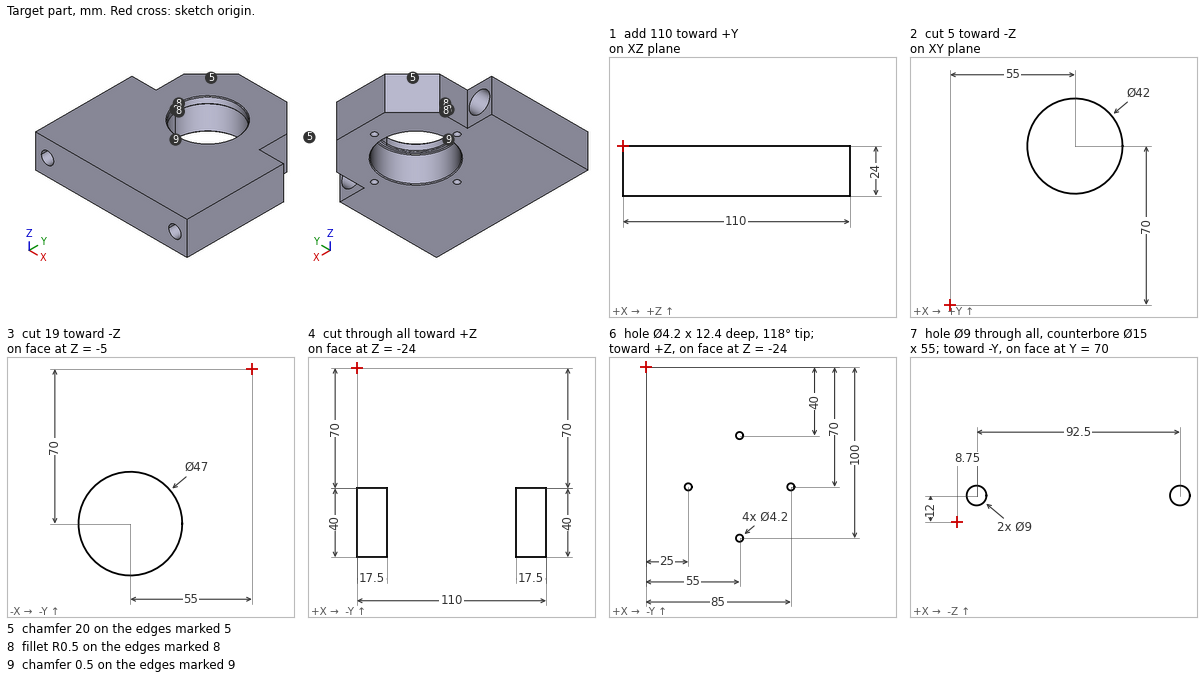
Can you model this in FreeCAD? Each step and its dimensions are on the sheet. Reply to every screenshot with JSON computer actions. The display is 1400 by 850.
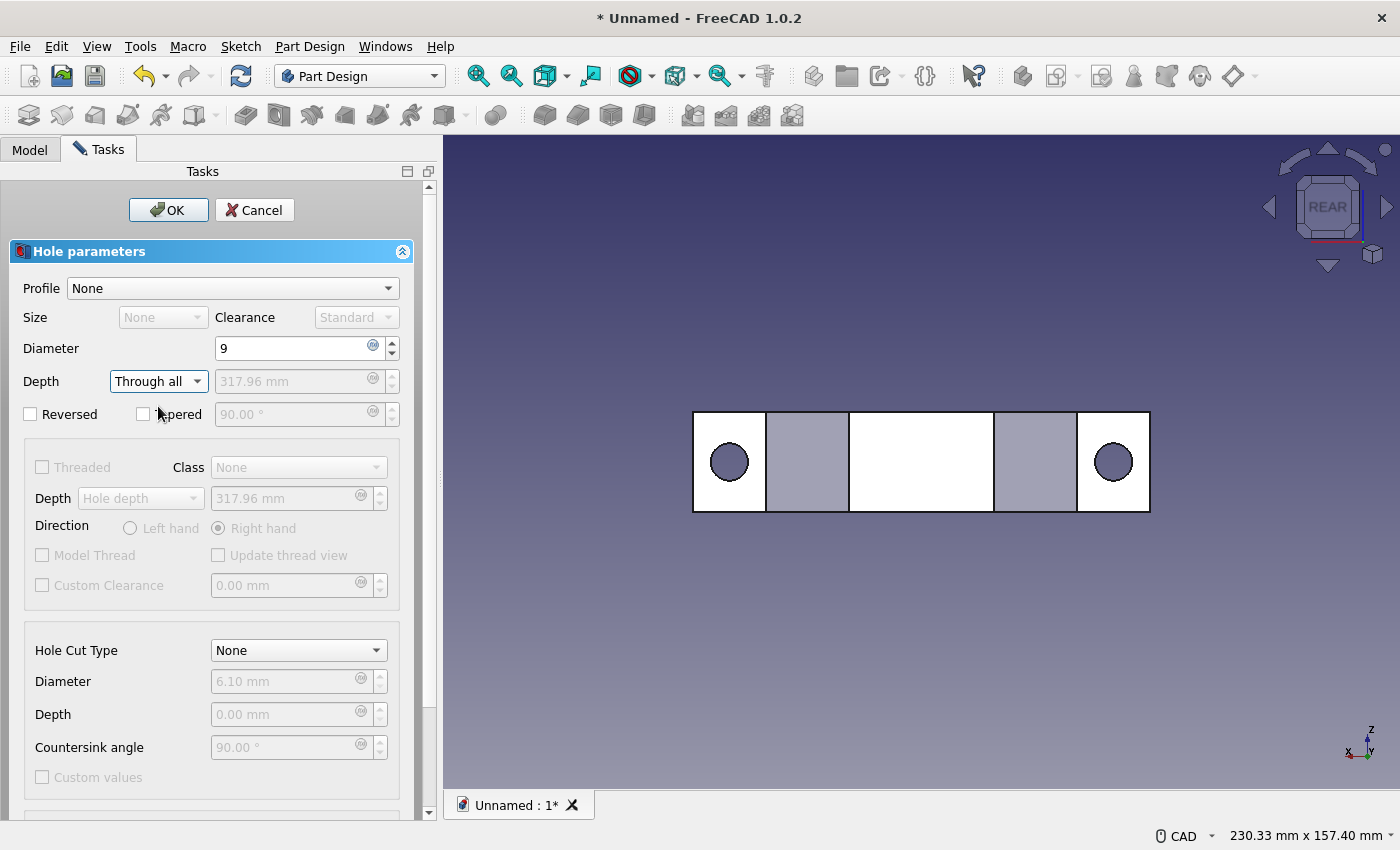
{"action": "left_click", "coordinate": [300, 650]}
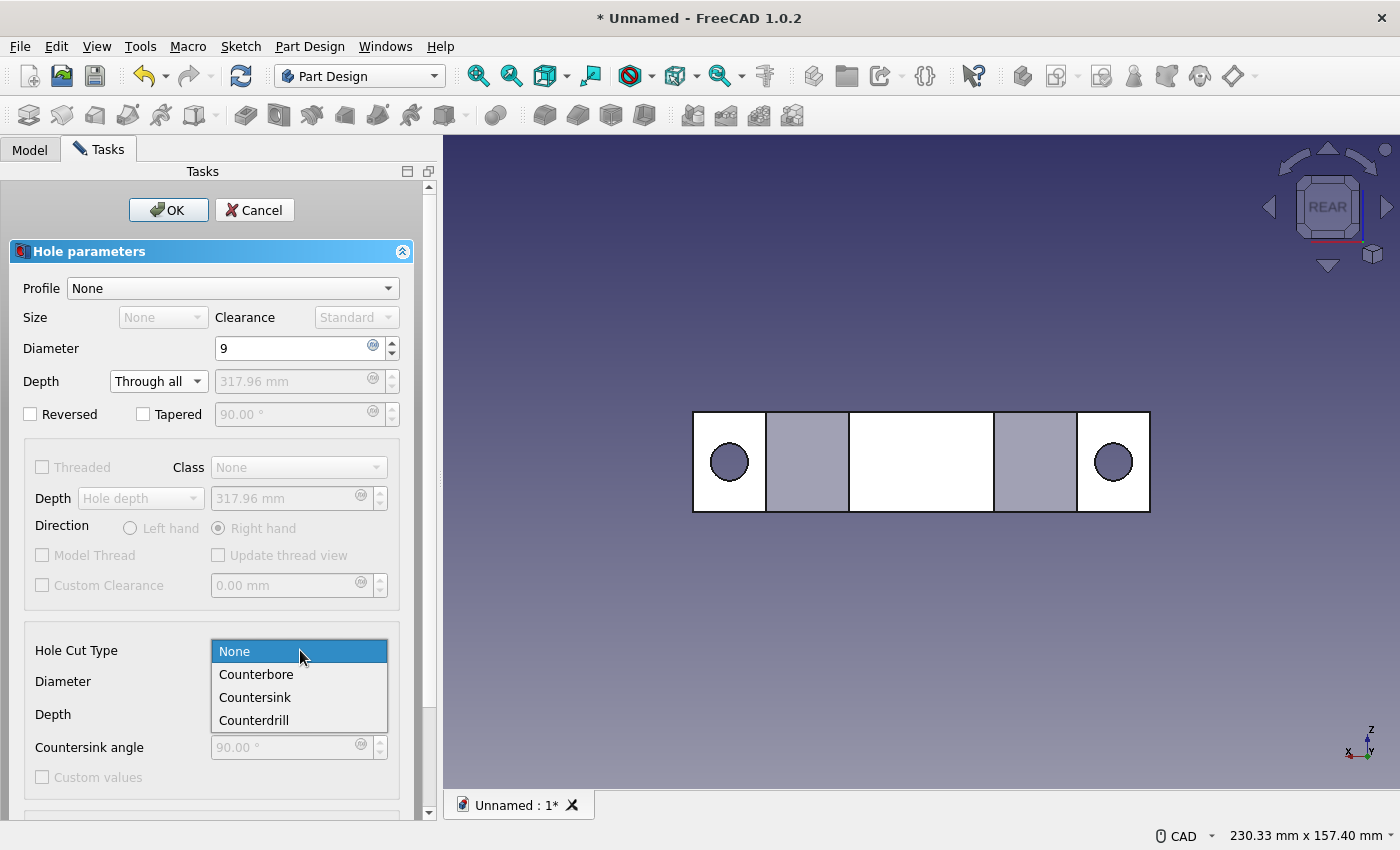
{"action": "left_click", "coordinate": [298, 674]}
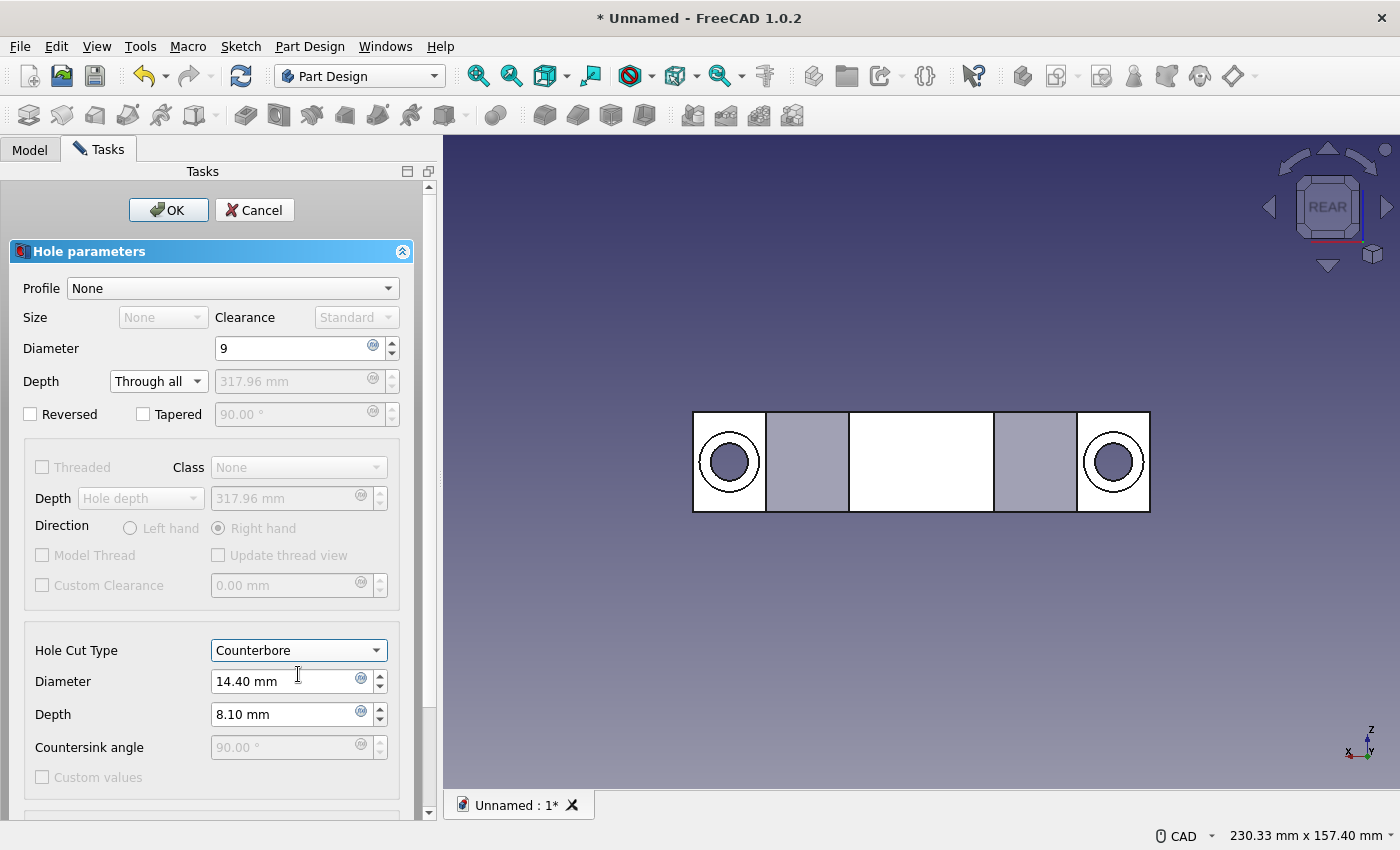
{"action": "triple_click", "coordinate": [292, 682]}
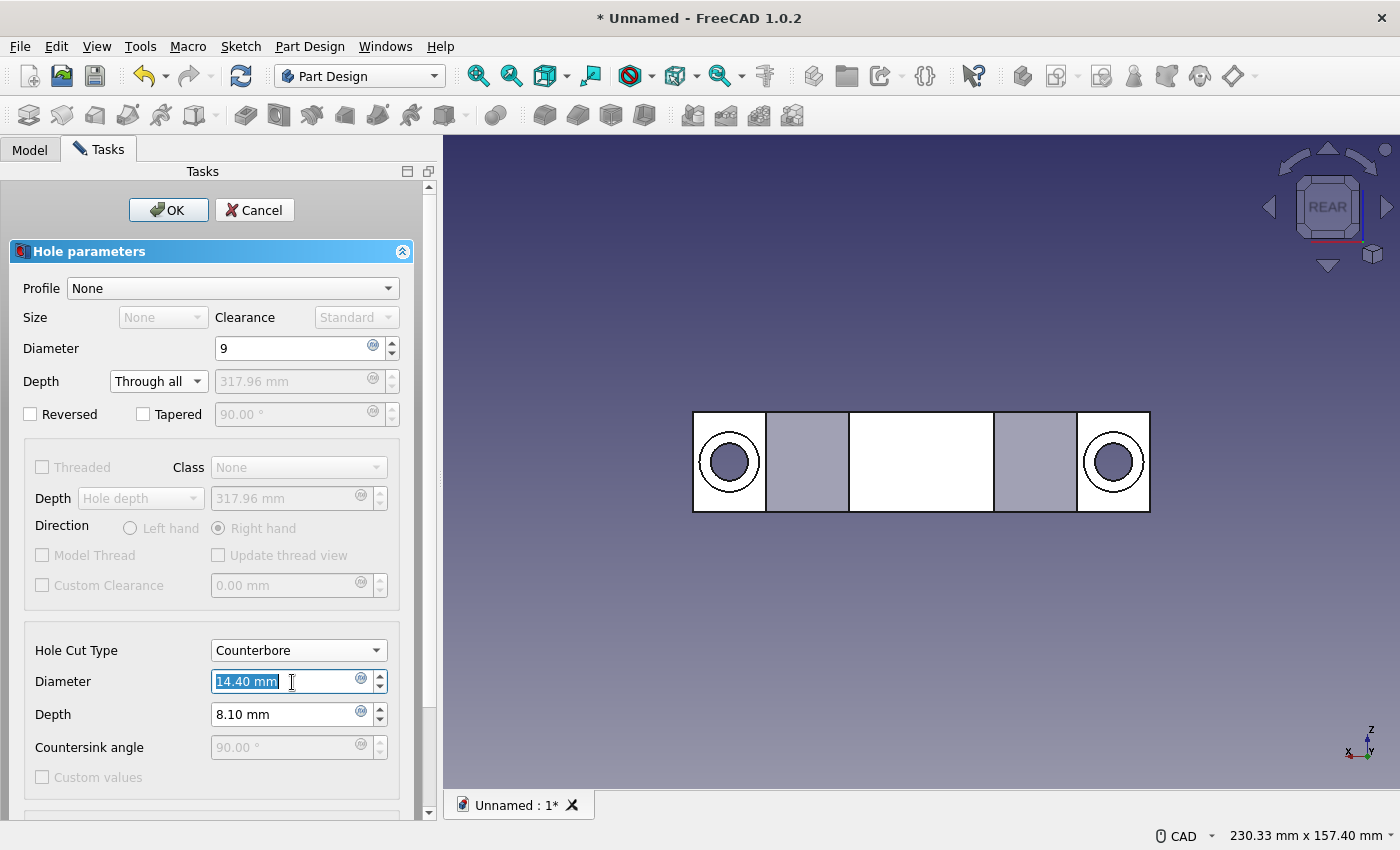
{"action": "type", "text": "15"}
{"action": "key", "text": "Tab"}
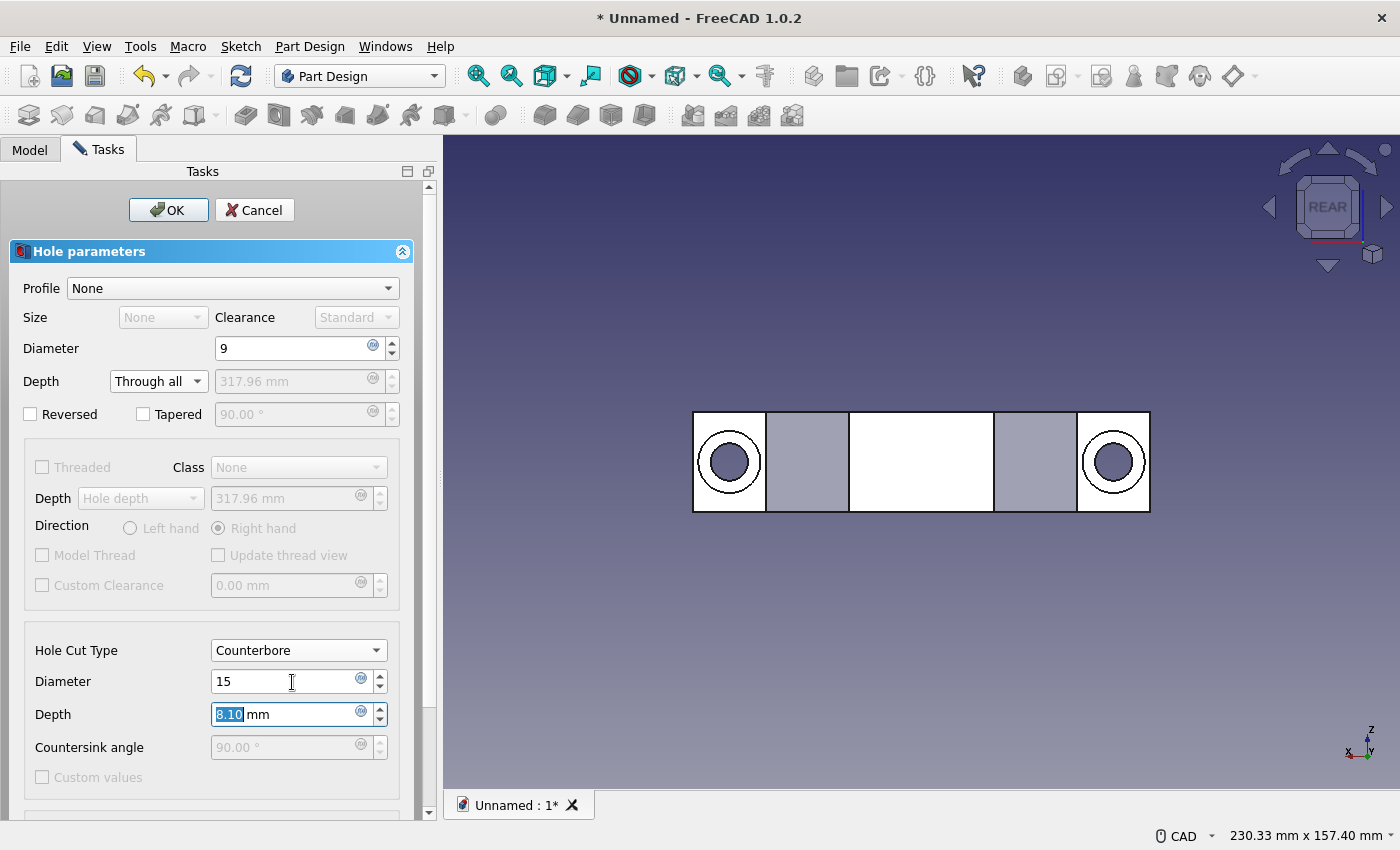
{"action": "type", "text": "55"}
{"action": "key", "text": "Tab"}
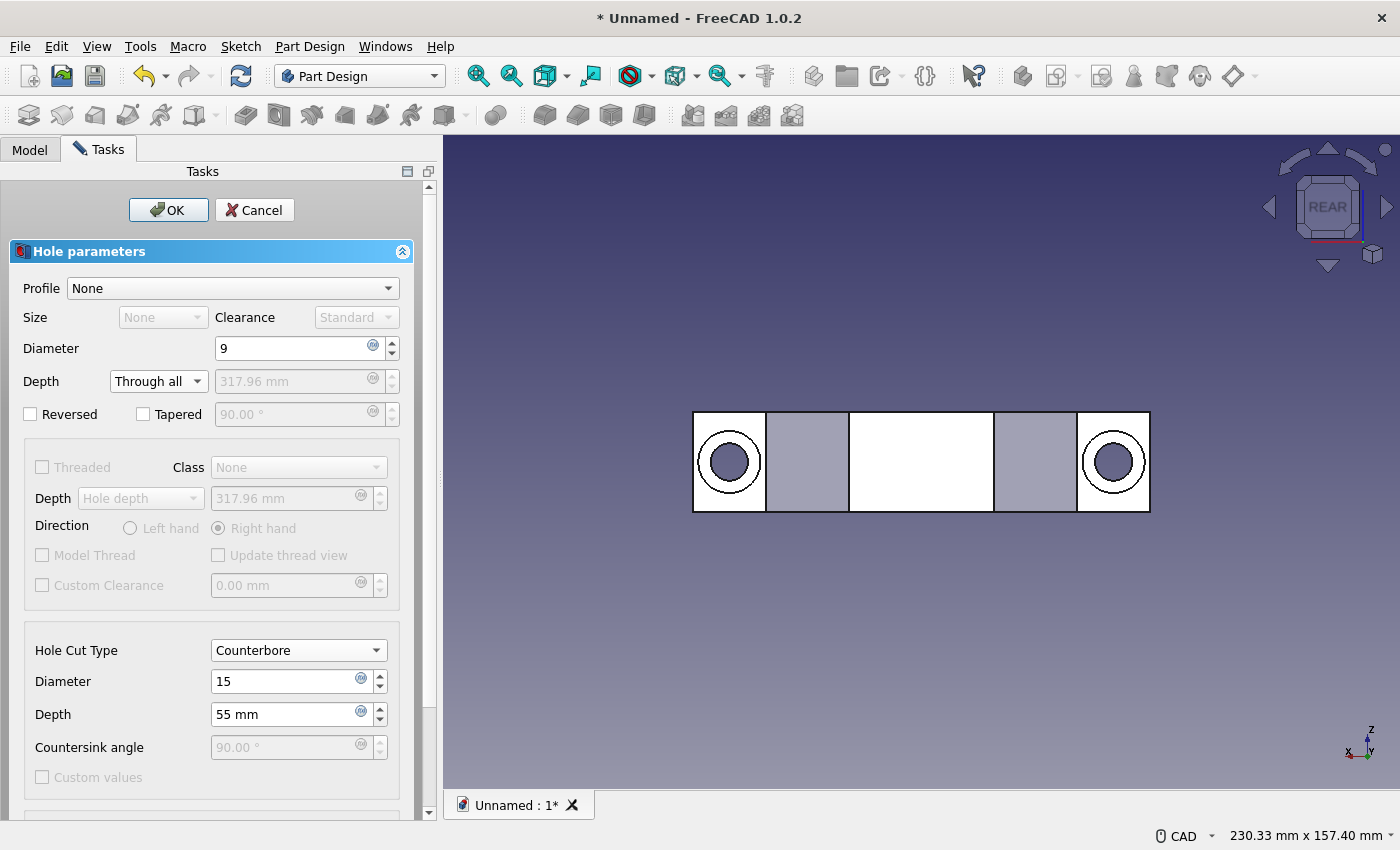
{"action": "left_click", "coordinate": [169, 210]}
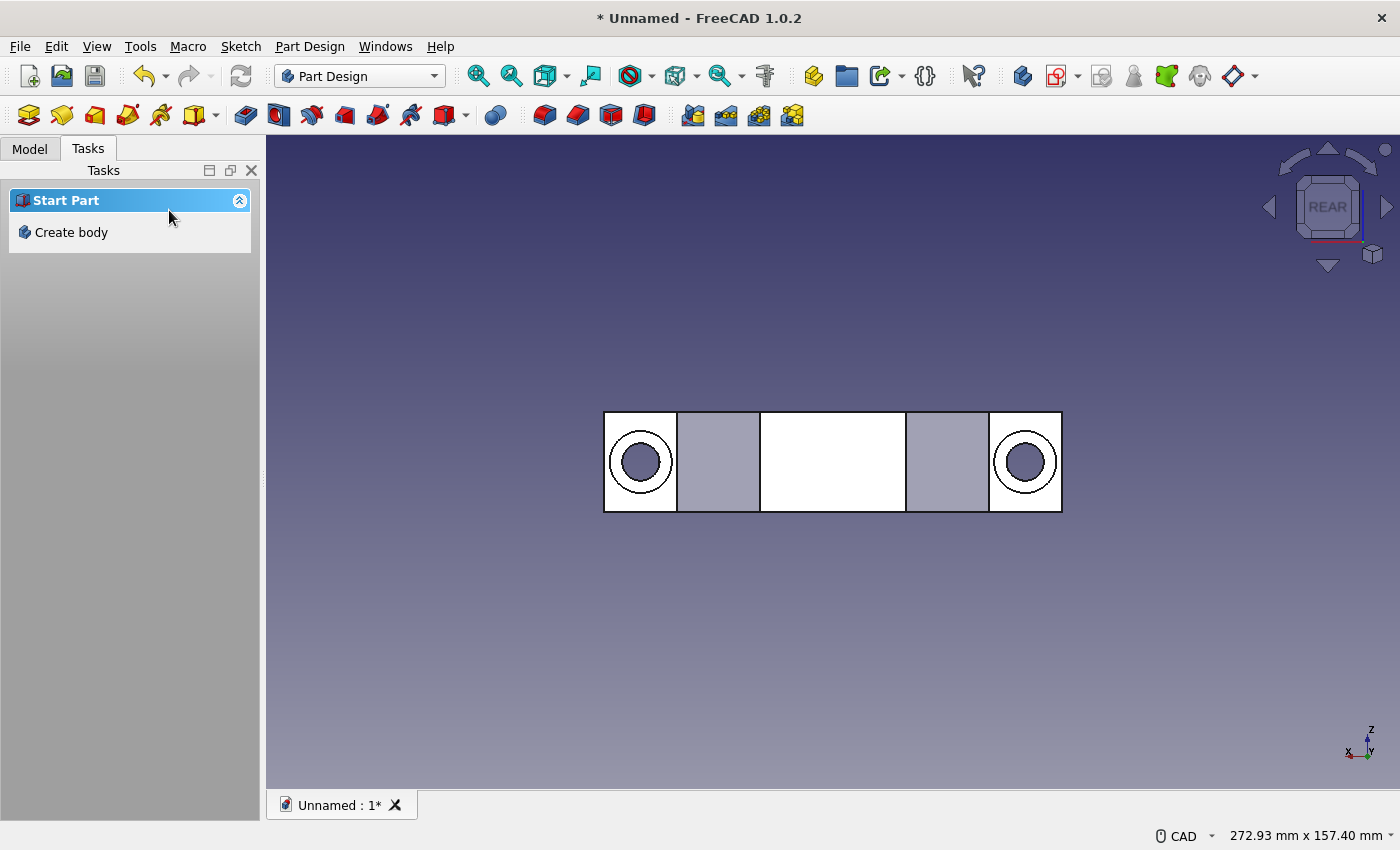
{"action": "key", "text": "v f"}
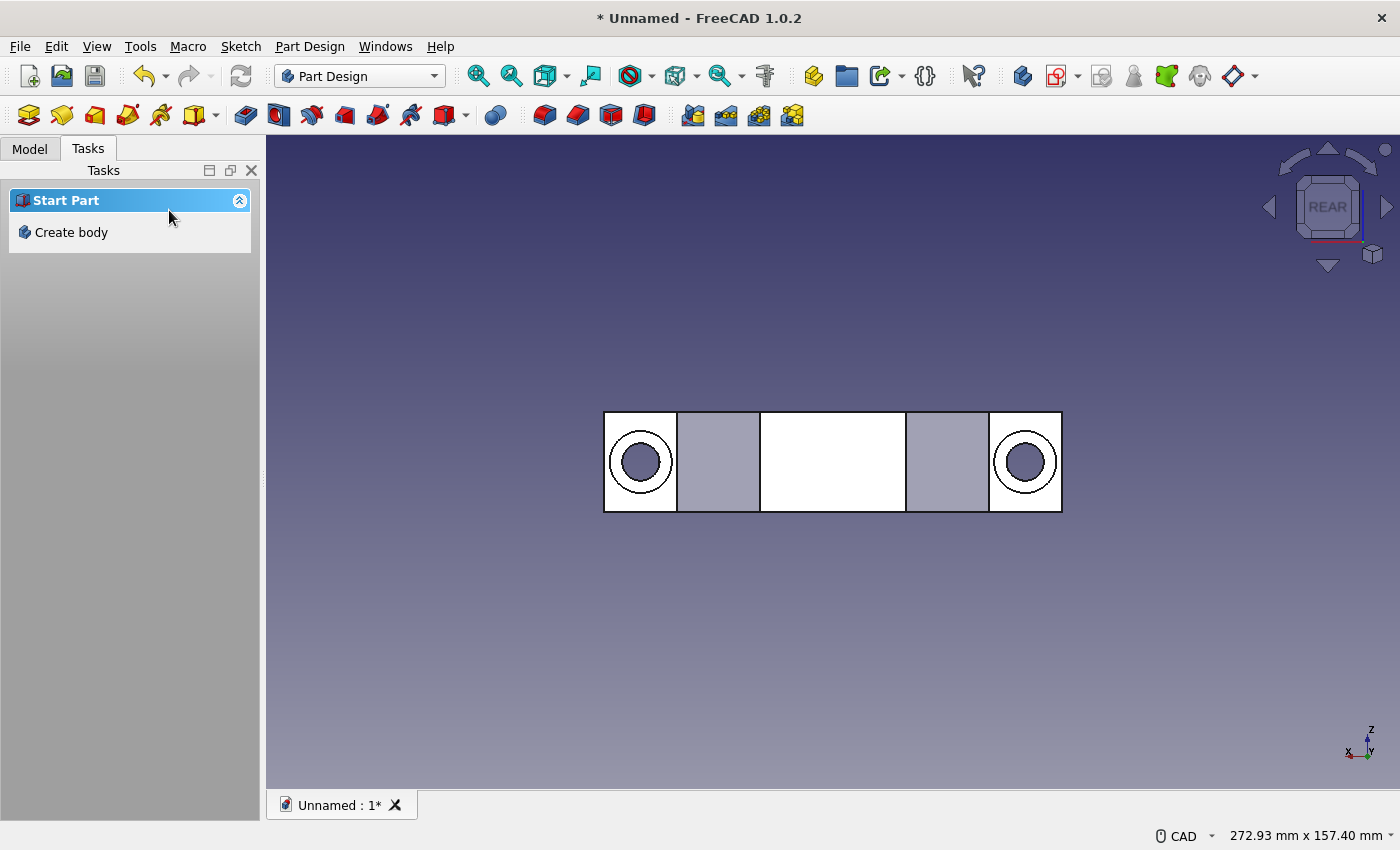
{"action": "key", "text": "0"}